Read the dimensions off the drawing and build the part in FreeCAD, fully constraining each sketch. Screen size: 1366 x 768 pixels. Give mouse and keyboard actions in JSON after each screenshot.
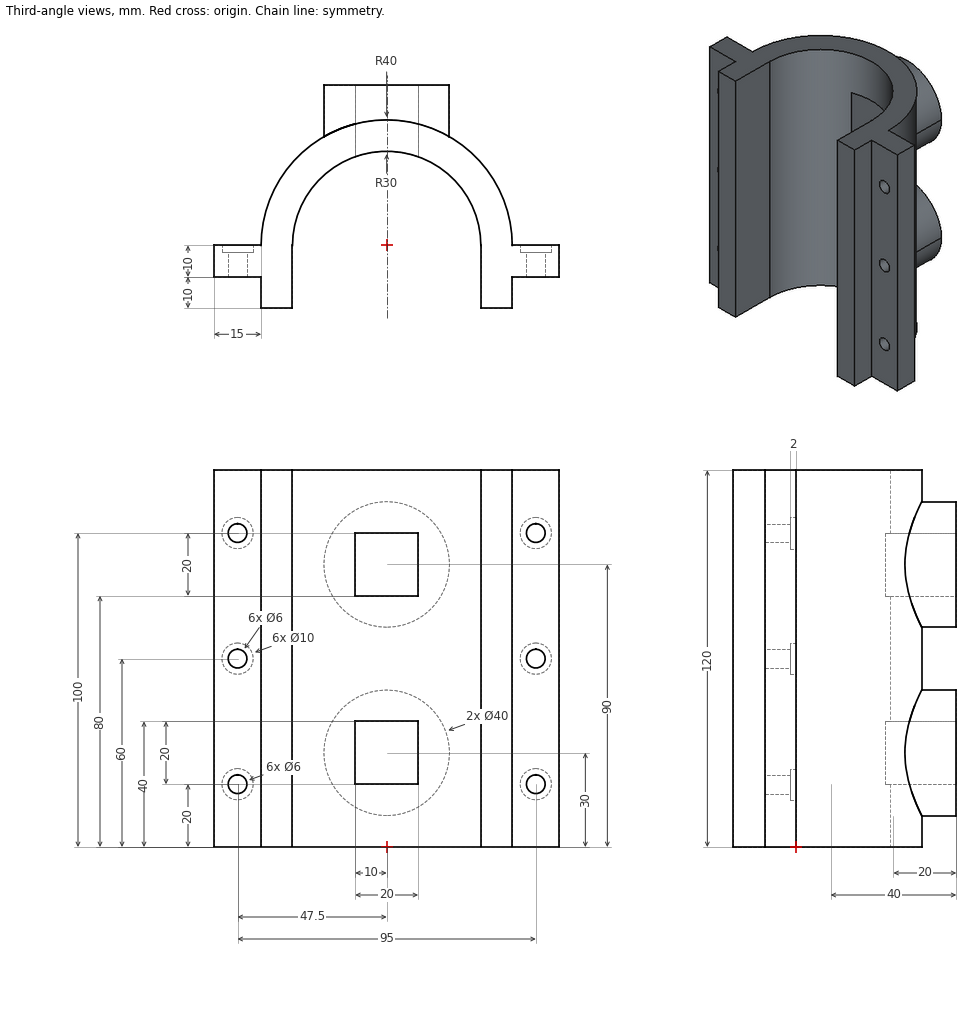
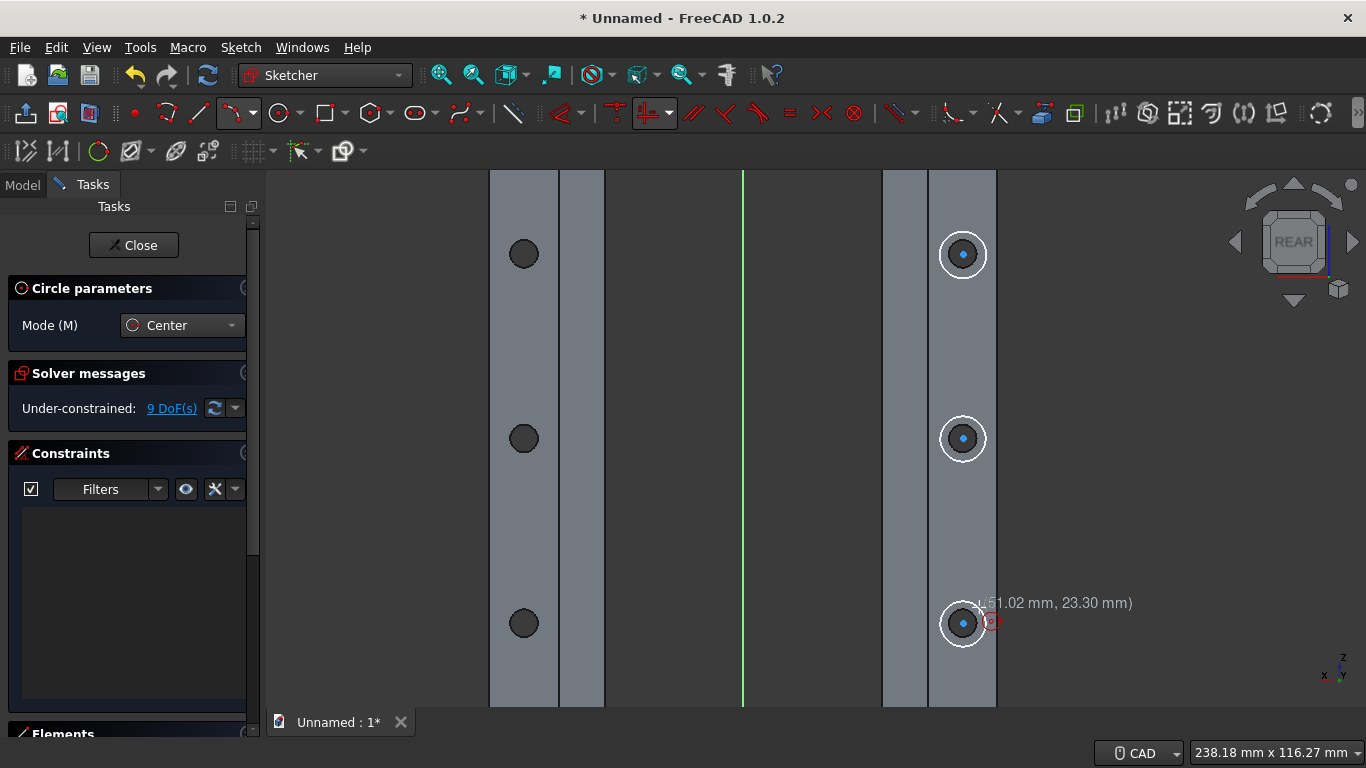
{"action": "left_click", "coordinate": [524, 623]}
{"action": "left_click", "coordinate": [540, 607]}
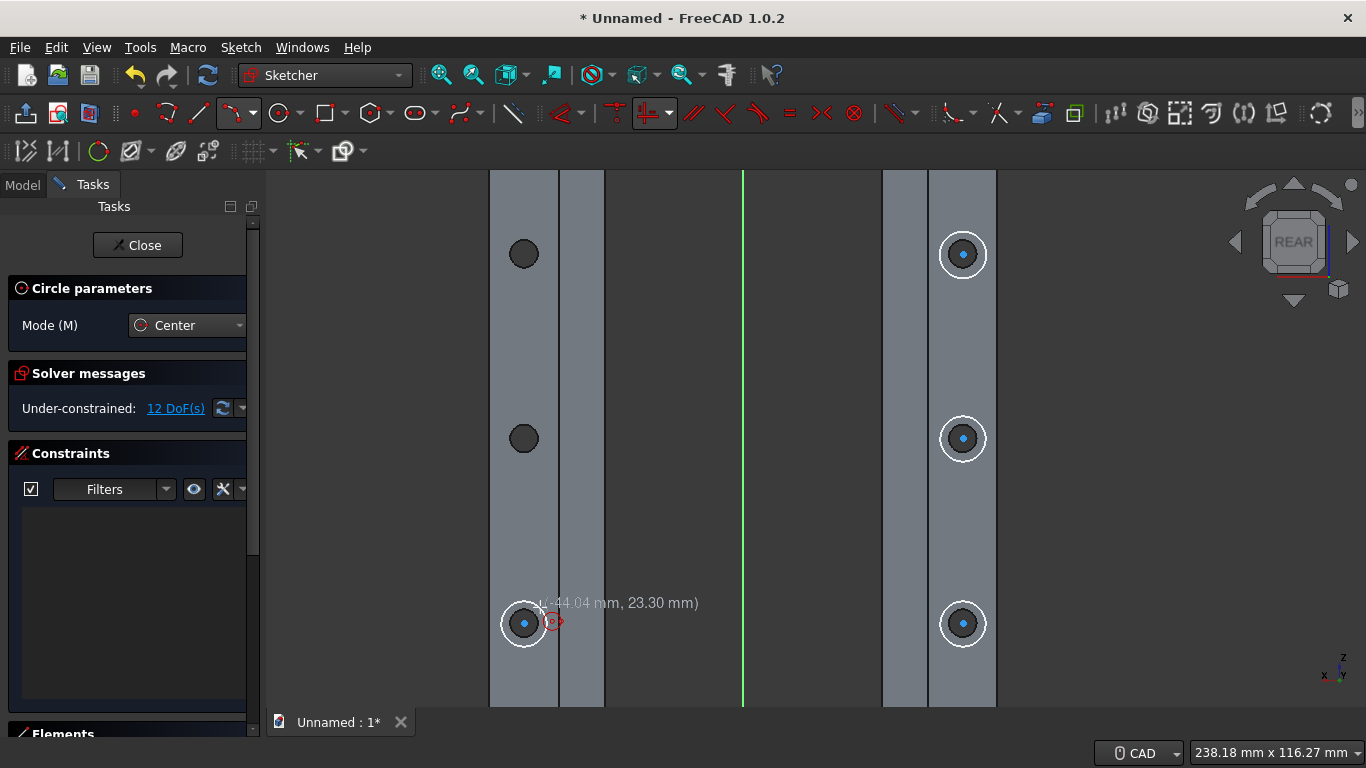
{"action": "left_click", "coordinate": [524, 438]}
{"action": "left_click", "coordinate": [540, 422]}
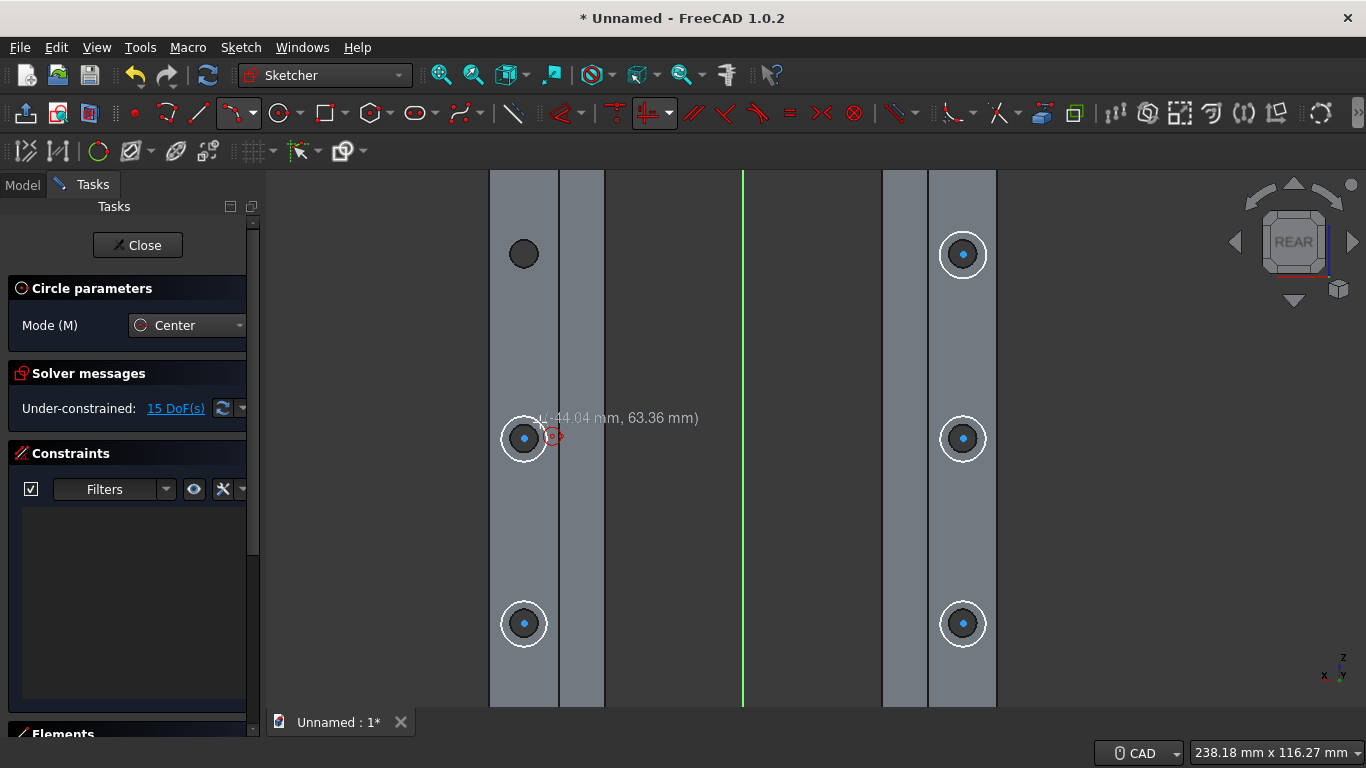
{"action": "left_click", "coordinate": [524, 254]}
{"action": "left_click", "coordinate": [540, 237]}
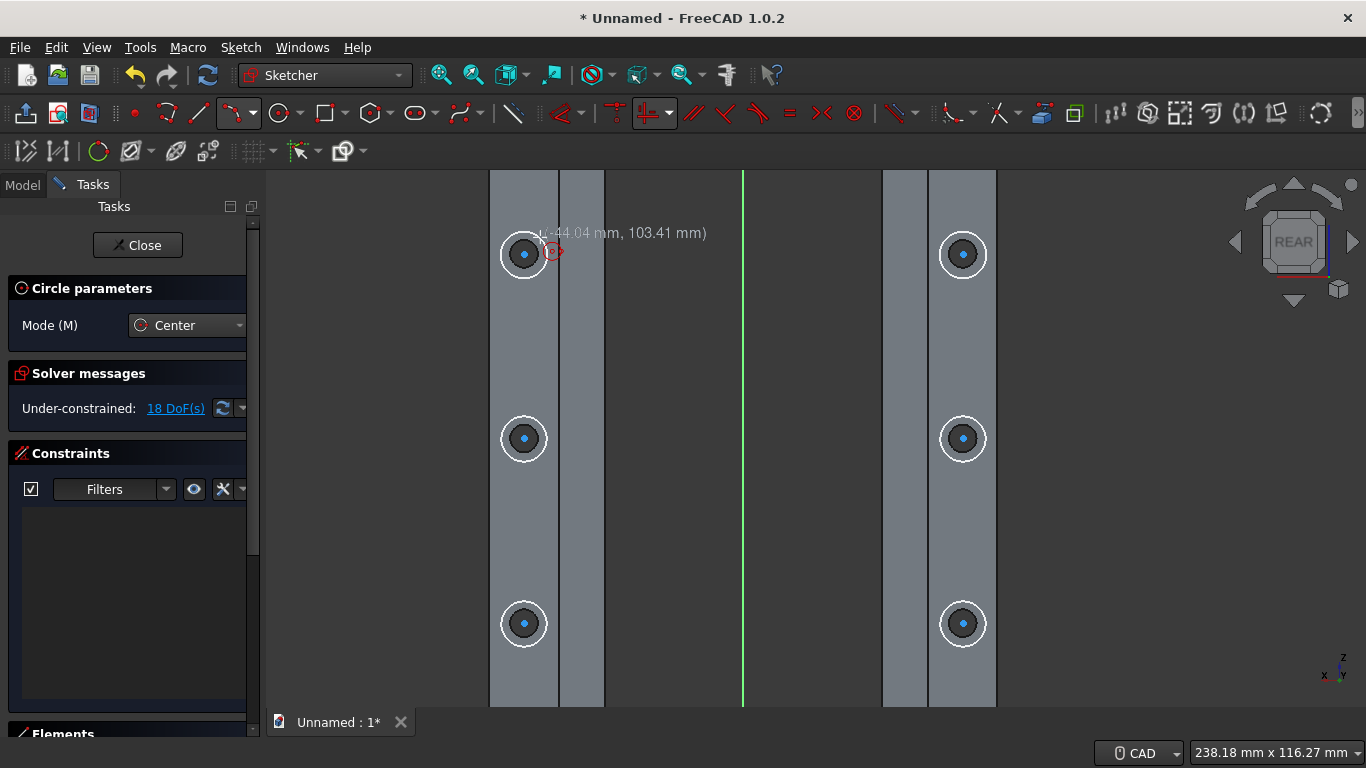
{"action": "scroll", "coordinate": [963, 438], "scroll_direction": "up", "scroll_amount": 3}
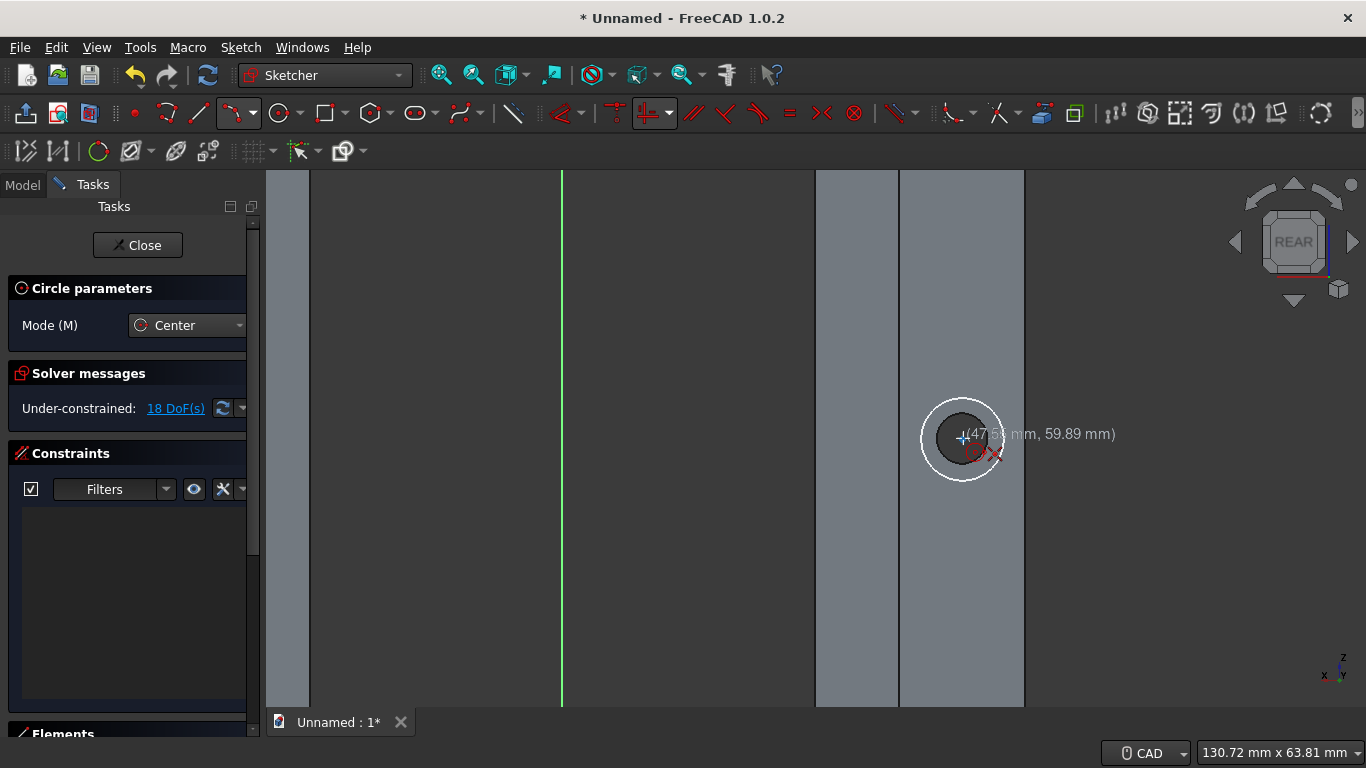
{"action": "left_click", "coordinate": [962, 439]}
{"action": "left_click", "coordinate": [980, 421]}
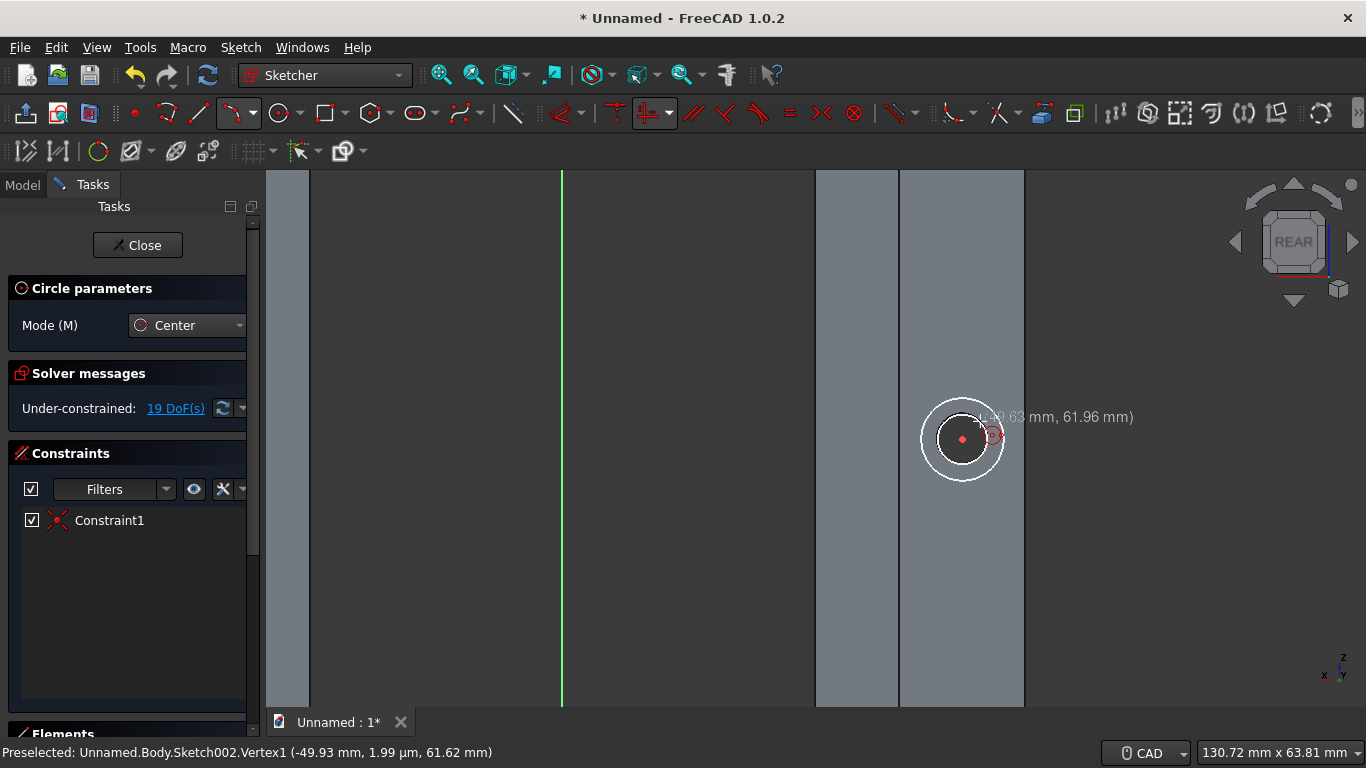
{"action": "scroll", "coordinate": [855, 402], "scroll_direction": "down", "scroll_amount": 5}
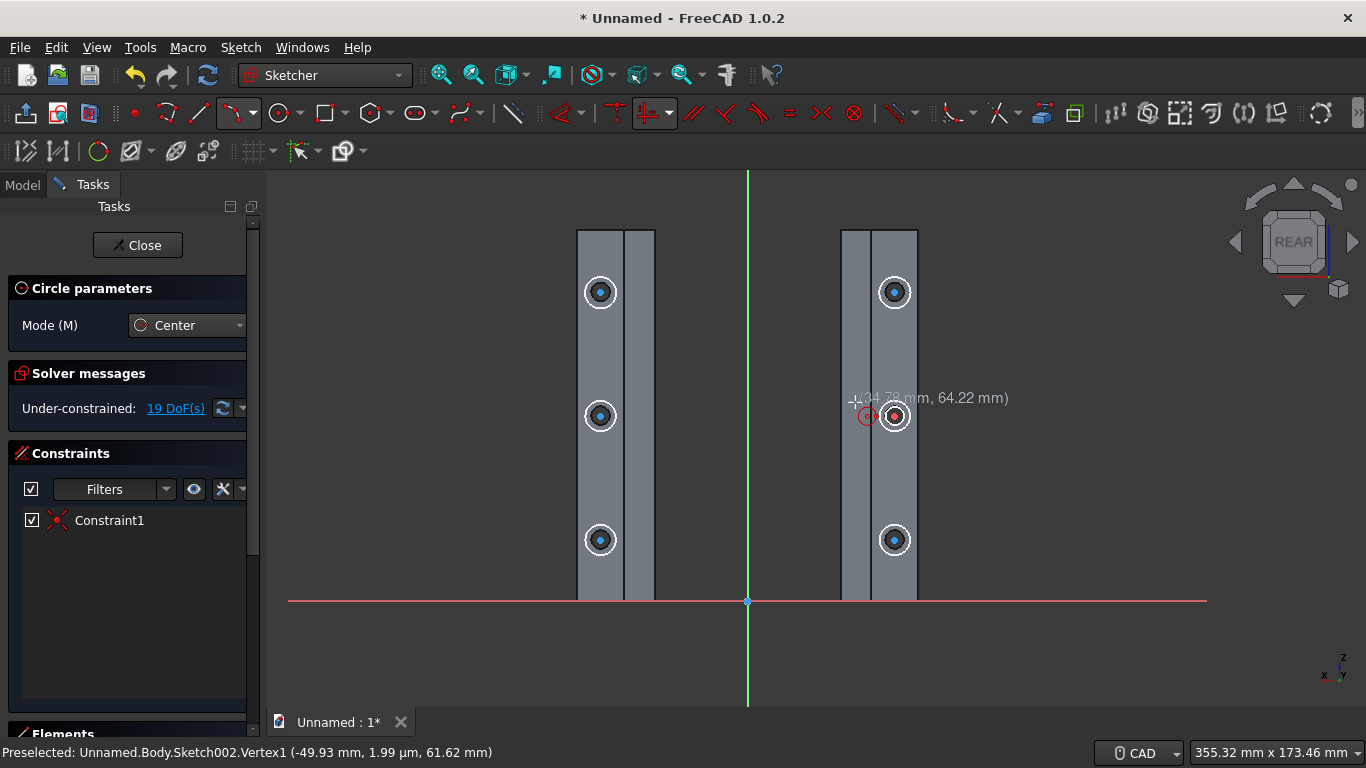
{"action": "scroll", "coordinate": [895, 292], "scroll_direction": "up", "scroll_amount": 5}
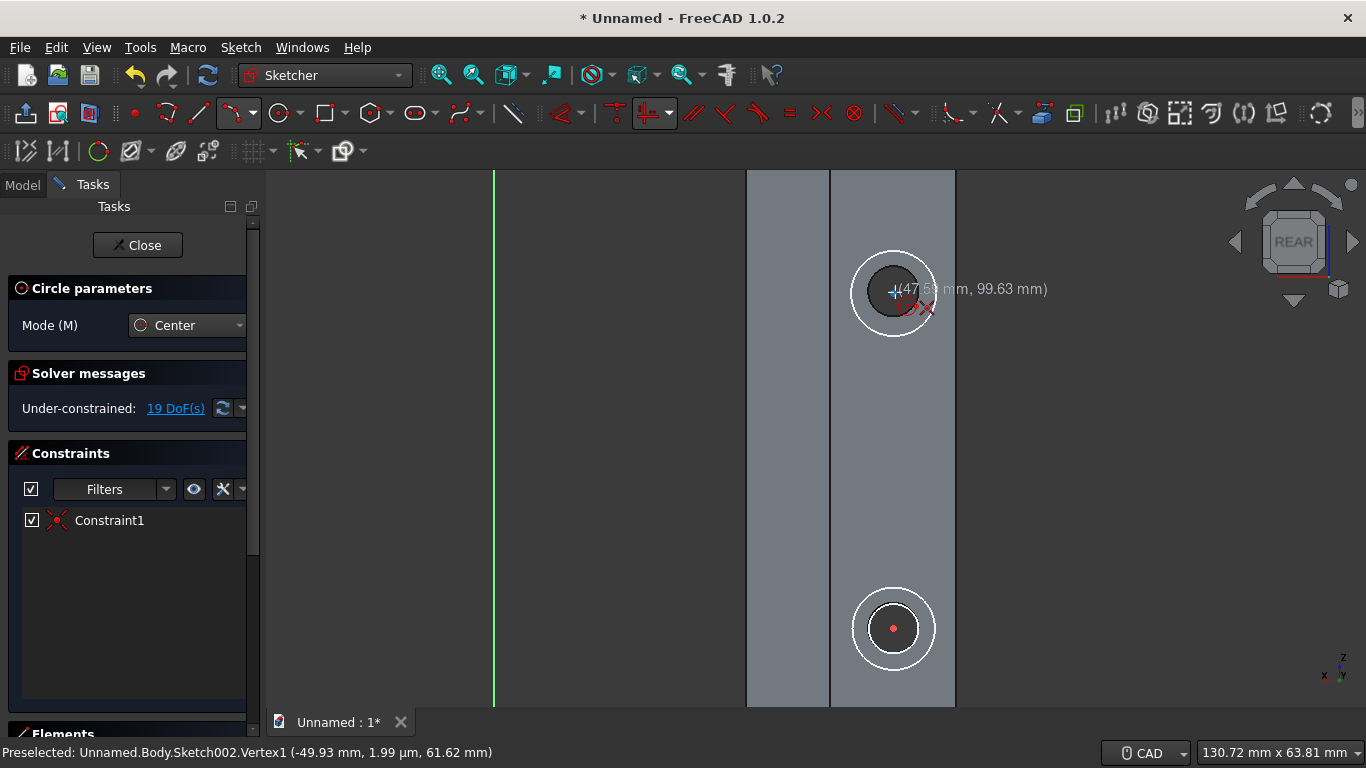
{"action": "left_click", "coordinate": [894, 294]}
{"action": "left_click", "coordinate": [911, 273]}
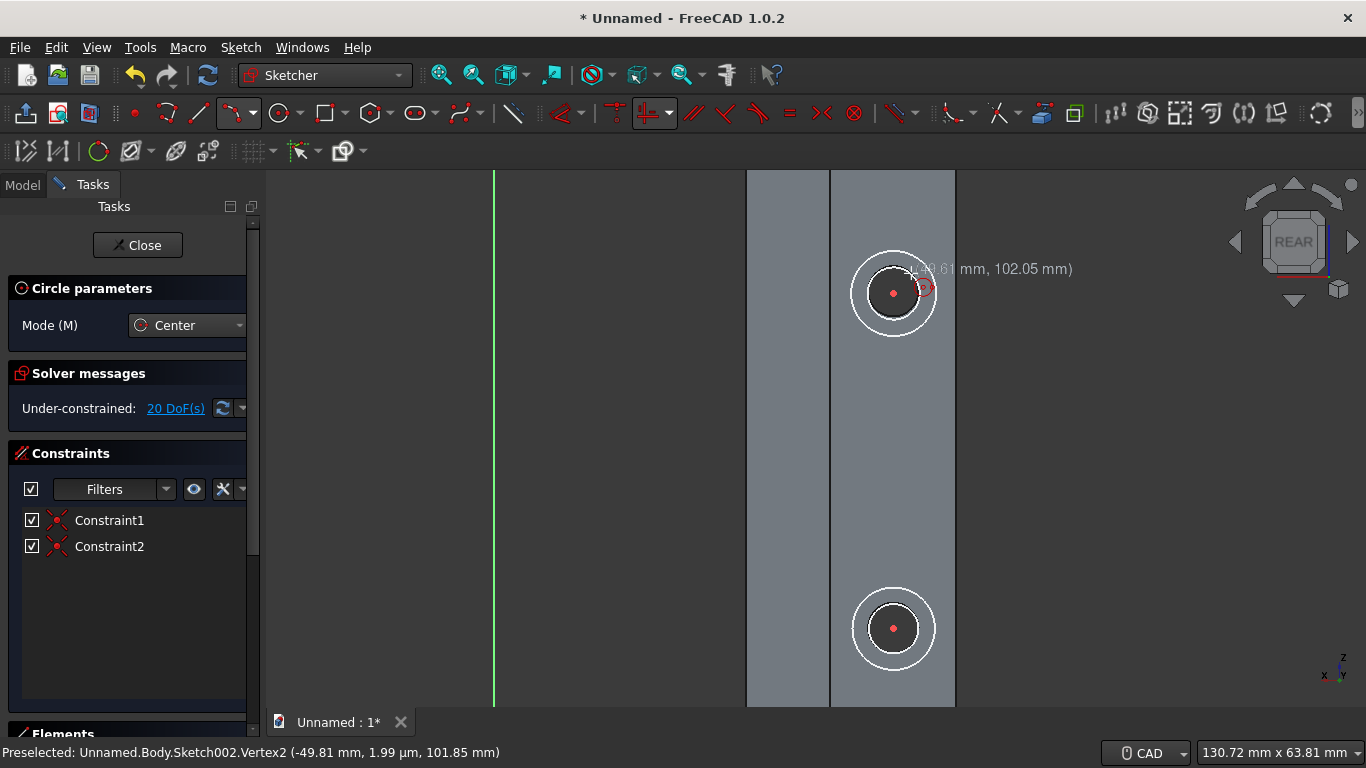
{"action": "scroll", "coordinate": [895, 292], "scroll_direction": "down", "scroll_amount": 5}